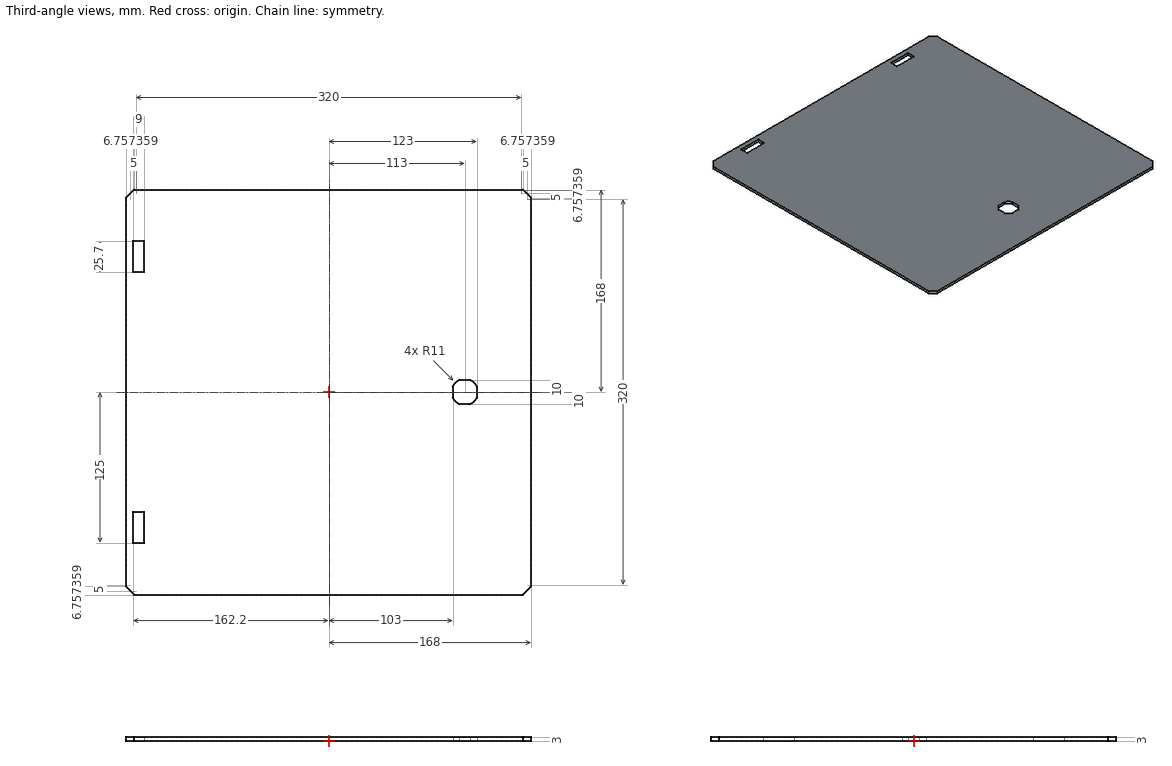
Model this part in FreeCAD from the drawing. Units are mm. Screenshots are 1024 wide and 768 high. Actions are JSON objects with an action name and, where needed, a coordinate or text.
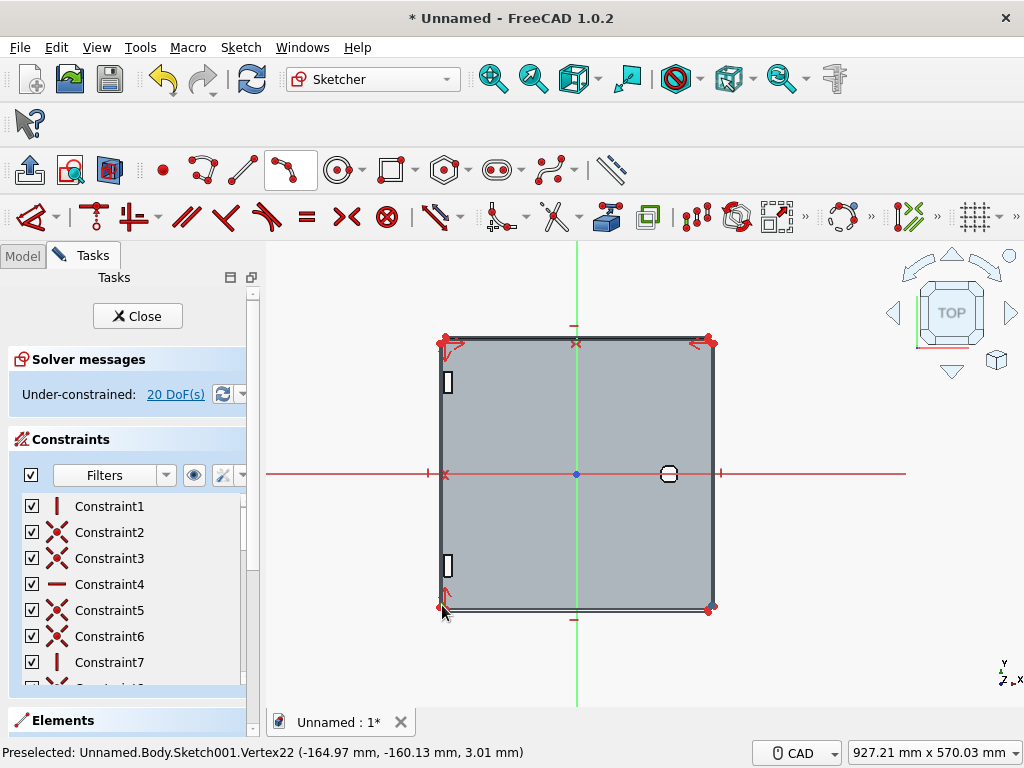
{"action": "left_click", "coordinate": [577, 650]}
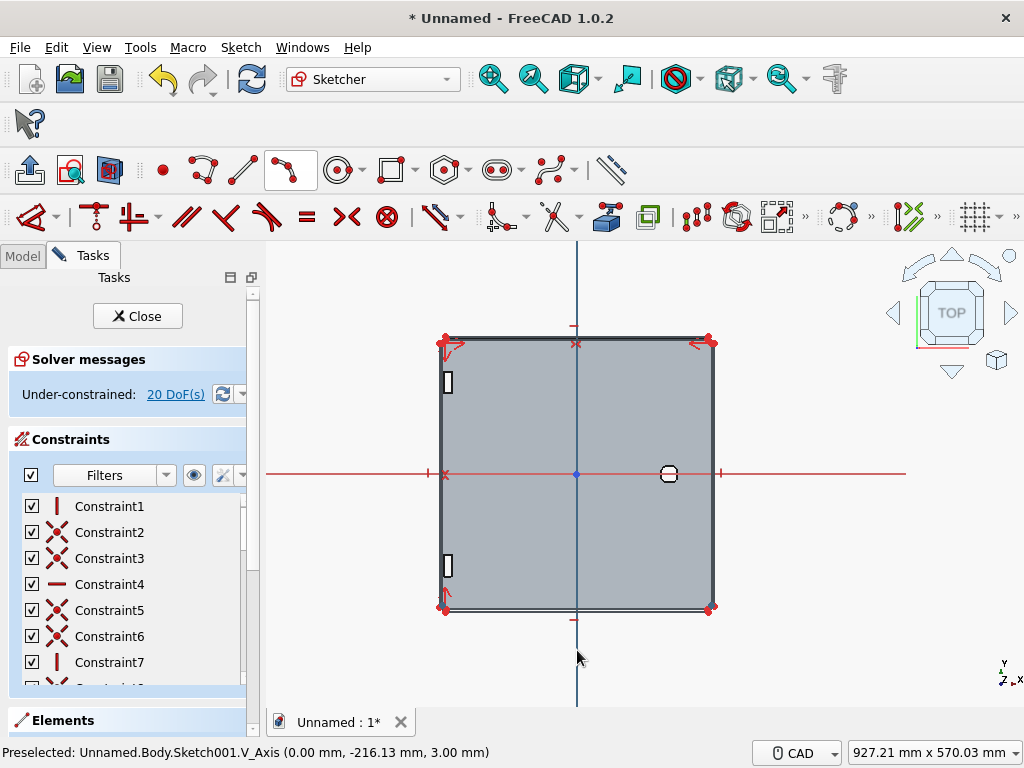
{"action": "left_click", "coordinate": [348, 218]}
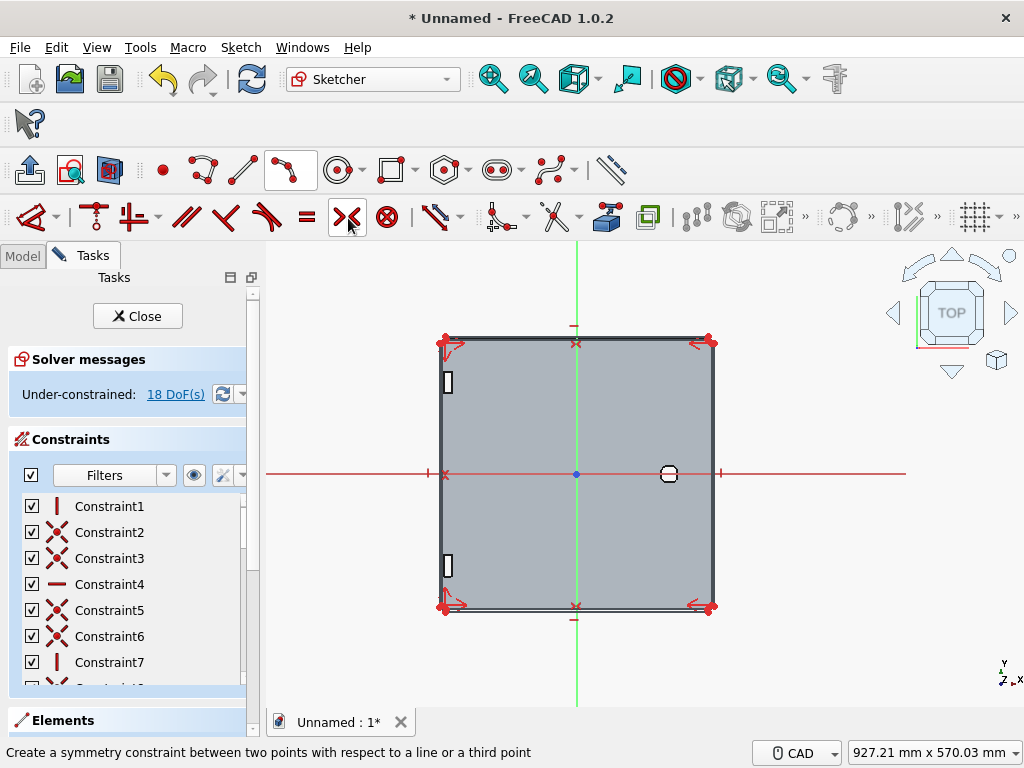
{"action": "scroll", "coordinate": [446, 609], "scroll_direction": "up", "scroll_amount": 8}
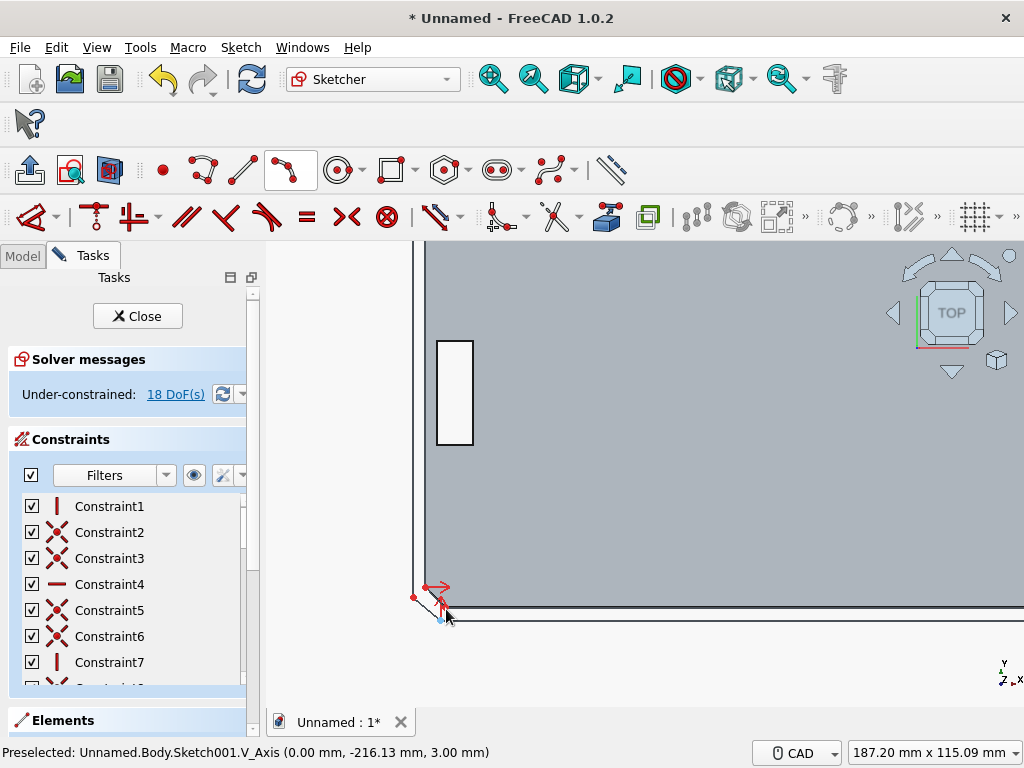
{"action": "left_click", "coordinate": [445, 608]}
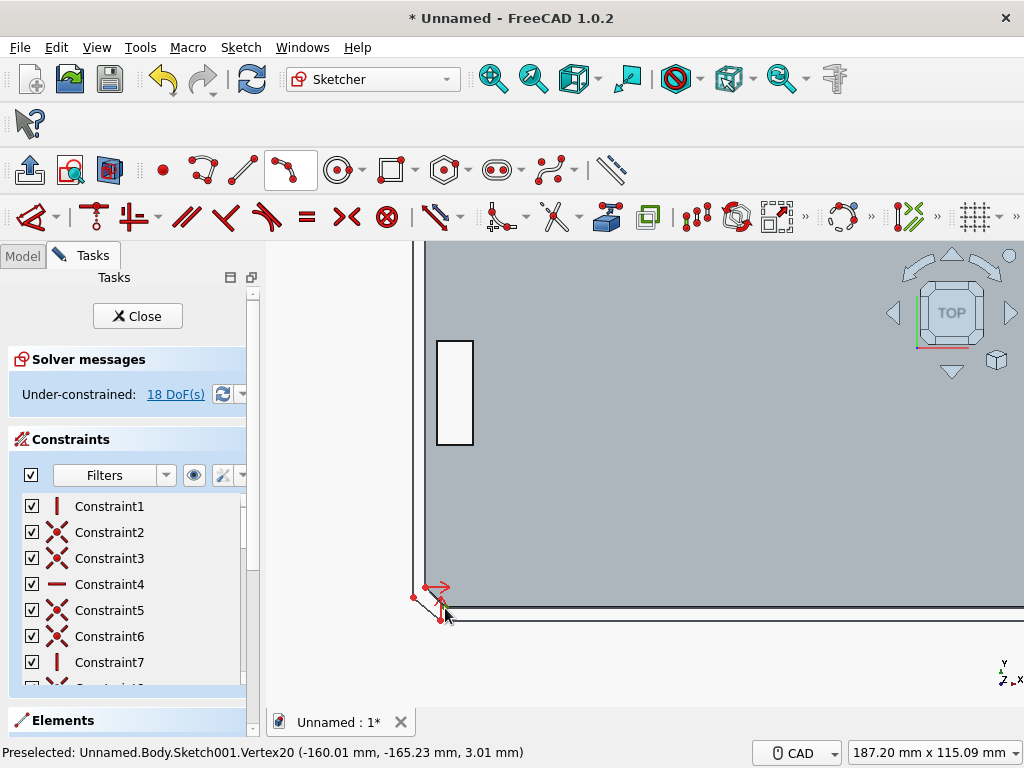
{"action": "scroll", "coordinate": [446, 609], "scroll_direction": "down", "scroll_amount": 8}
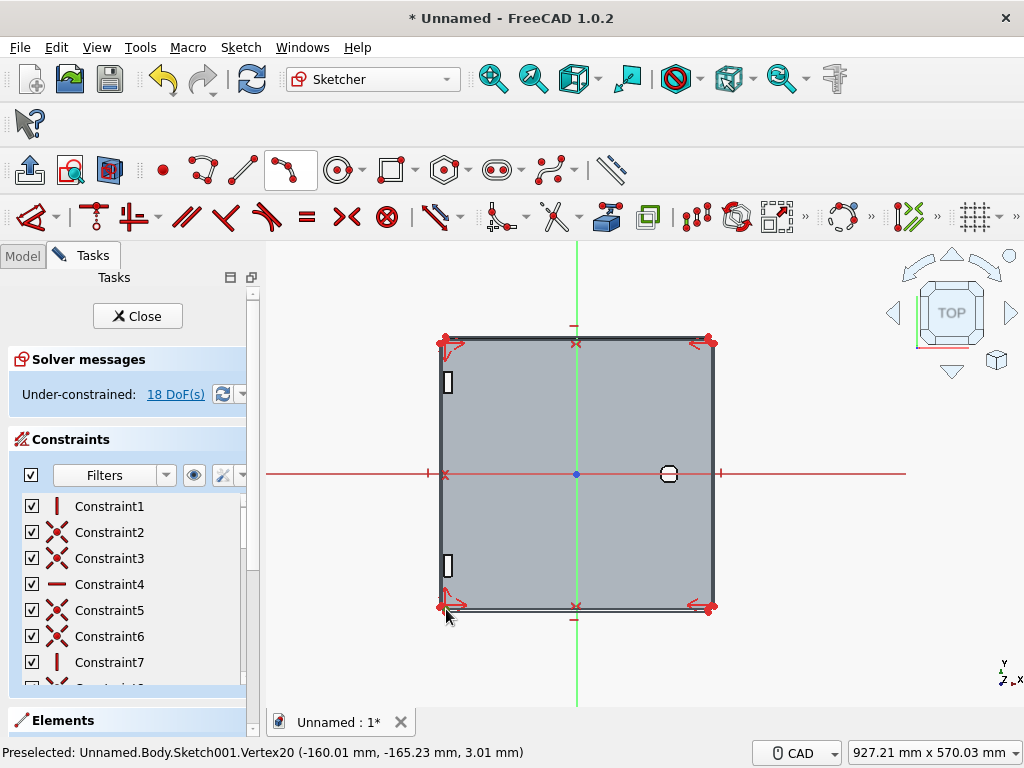
{"action": "scroll", "coordinate": [446, 340], "scroll_direction": "up", "scroll_amount": 7}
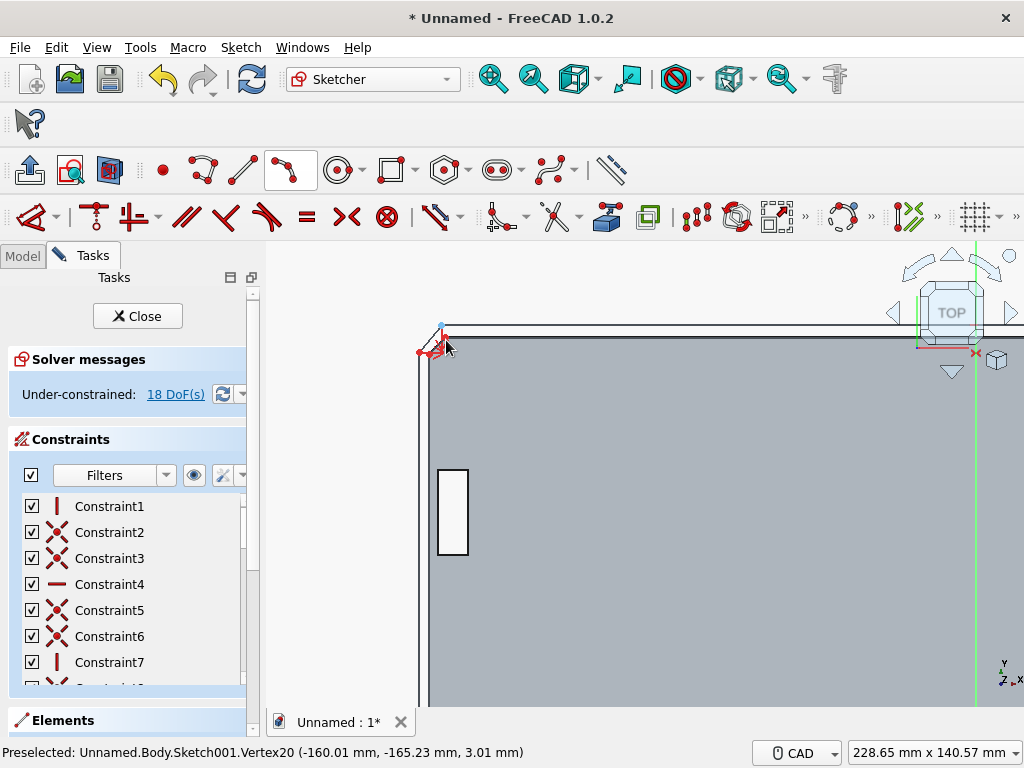
{"action": "left_click", "coordinate": [446, 338]}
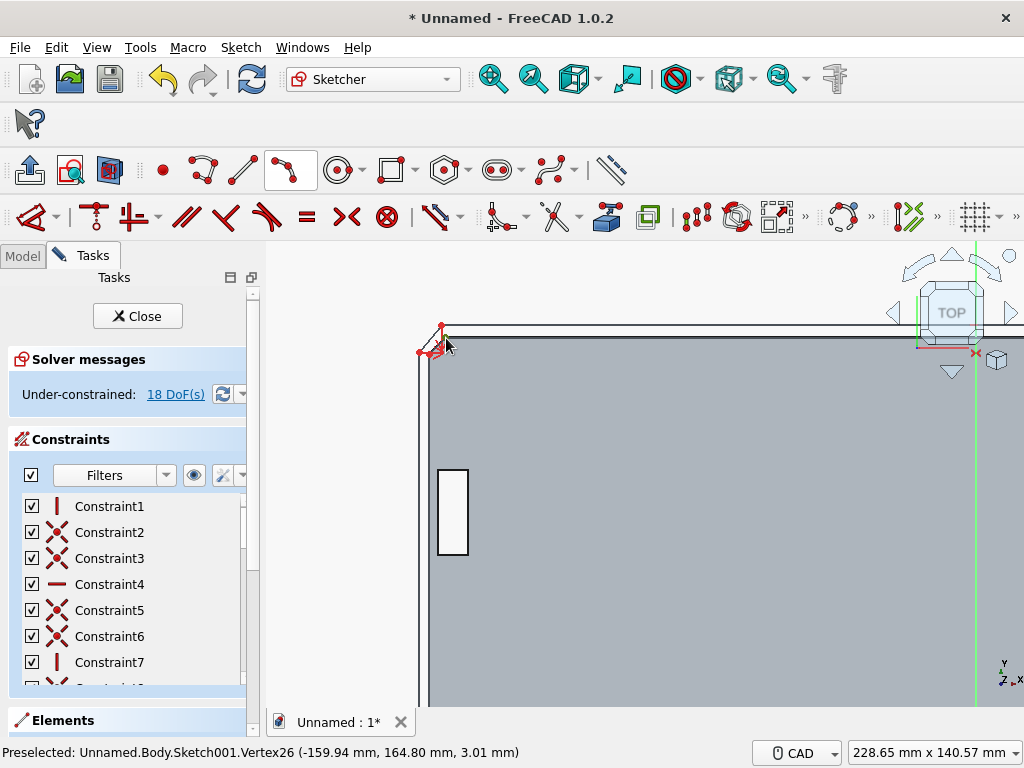
{"action": "scroll", "coordinate": [446, 340], "scroll_direction": "down", "scroll_amount": 7}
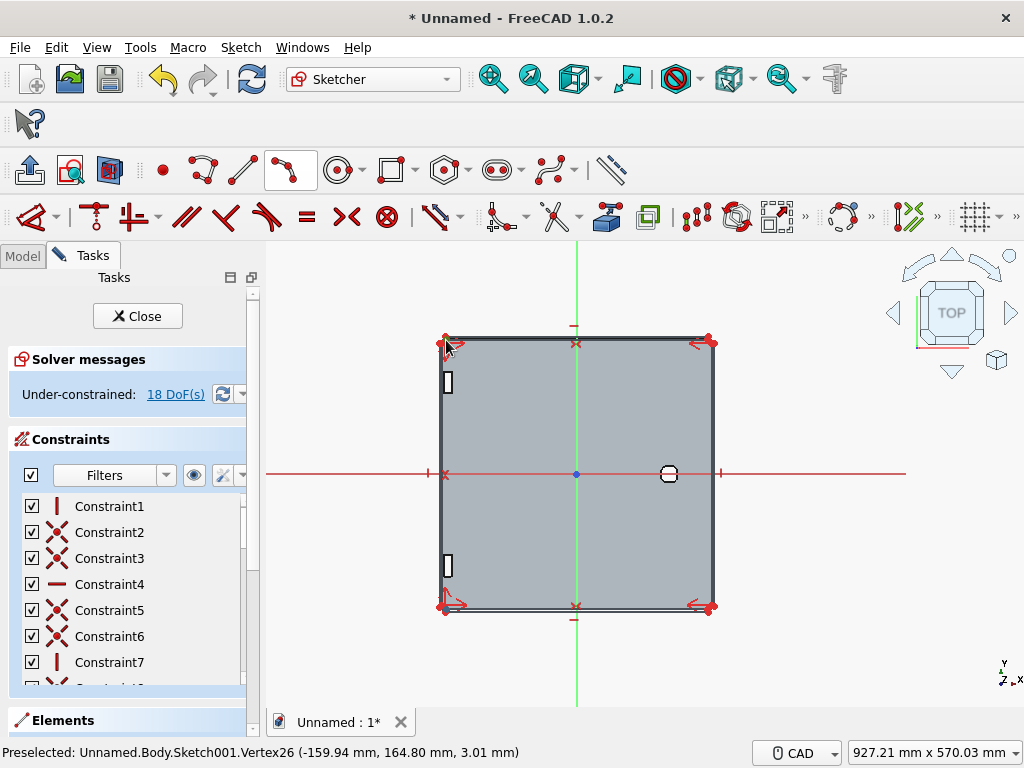
{"action": "left_click", "coordinate": [334, 474]}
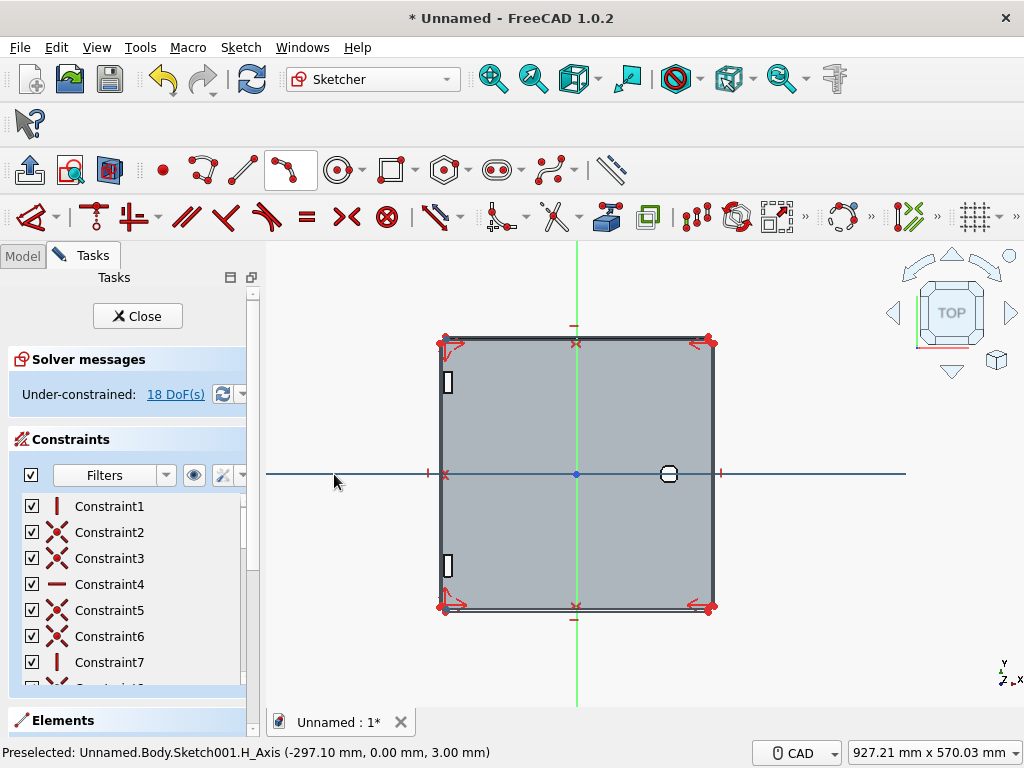
{"action": "left_click", "coordinate": [348, 218]}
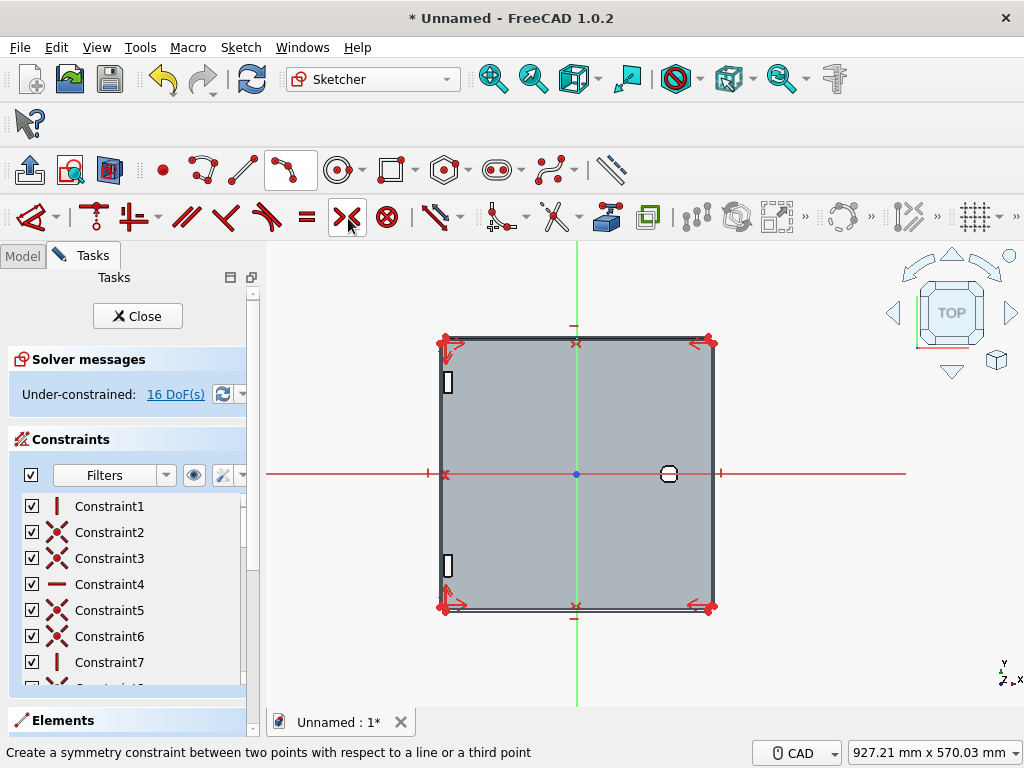
{"action": "left_click", "coordinate": [32, 218]}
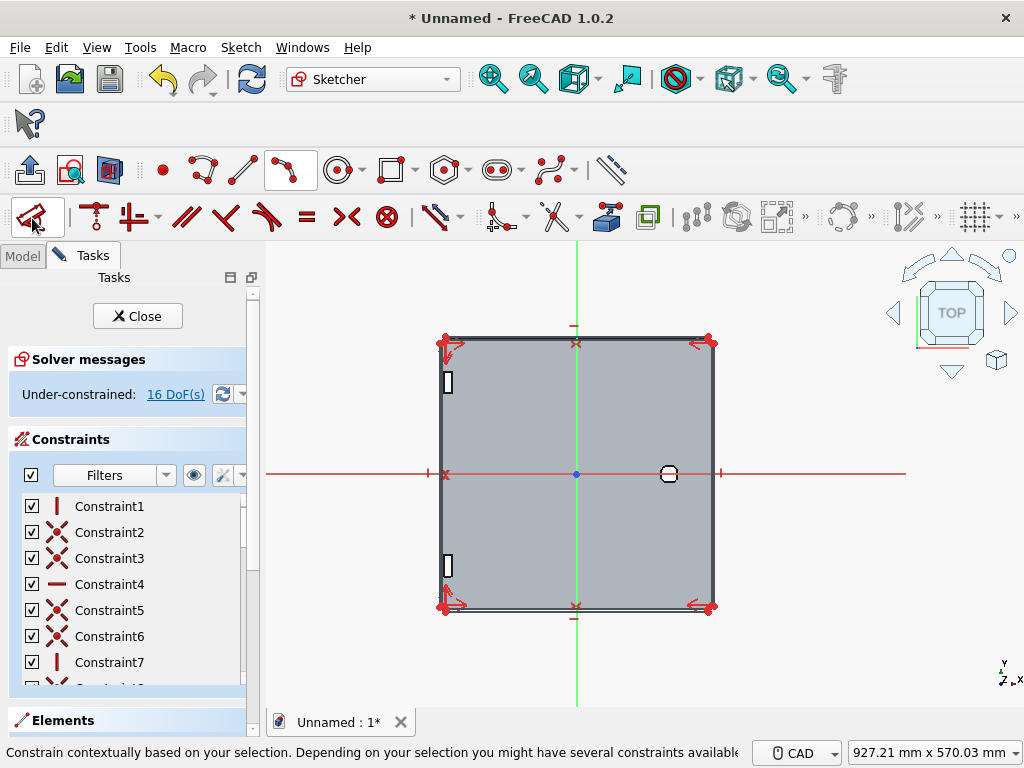
{"action": "scroll", "coordinate": [710, 607], "scroll_direction": "up", "scroll_amount": 12}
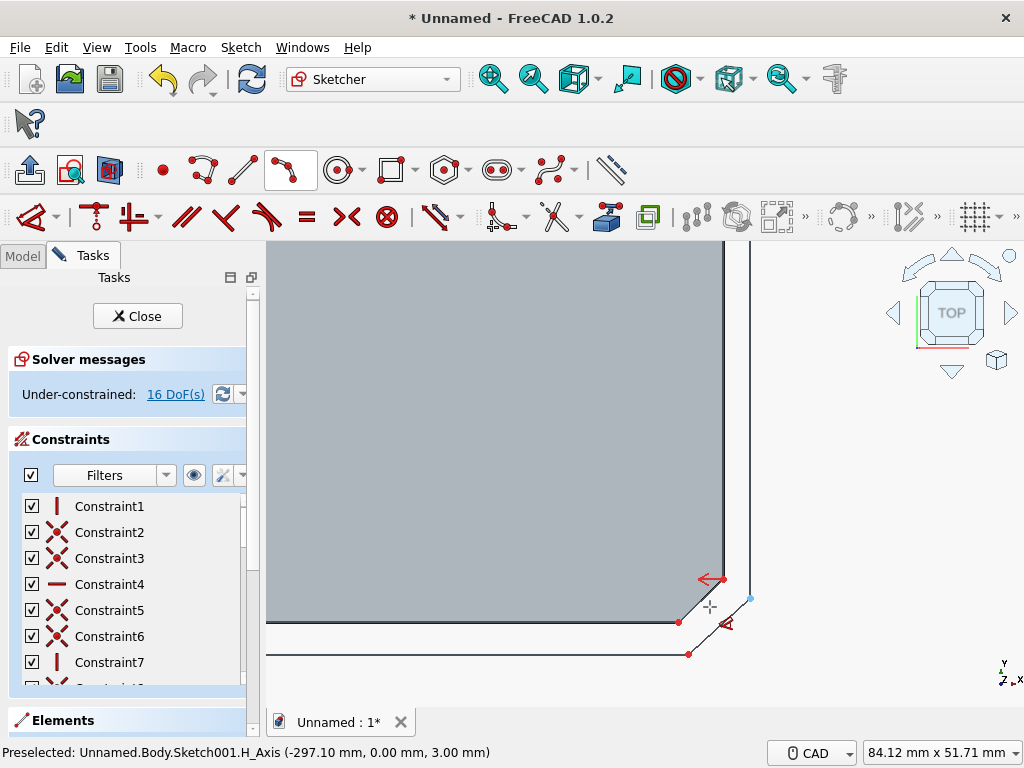
{"action": "left_click", "coordinate": [701, 601]}
{"action": "left_click", "coordinate": [711, 656]}